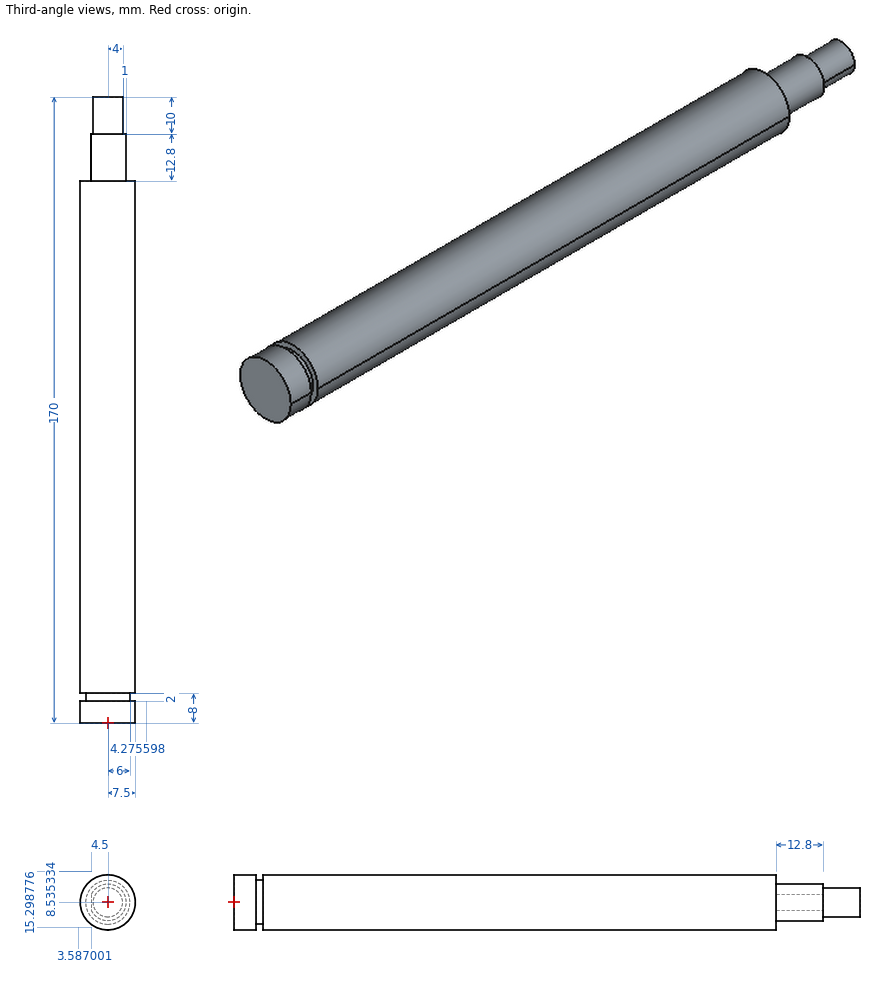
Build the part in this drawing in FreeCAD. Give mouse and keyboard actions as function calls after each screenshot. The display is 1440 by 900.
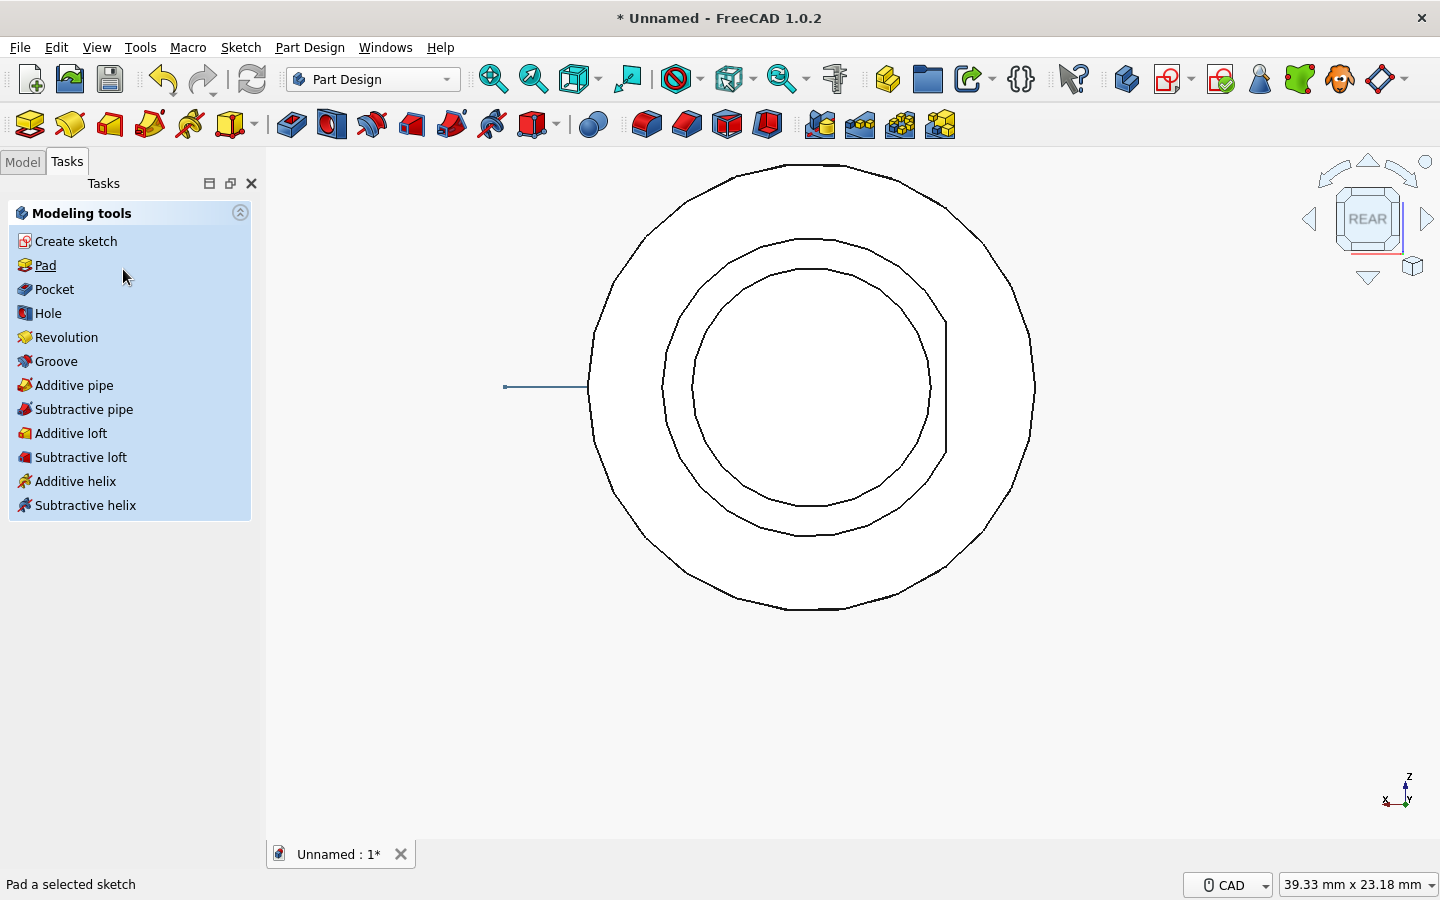
click(372, 124)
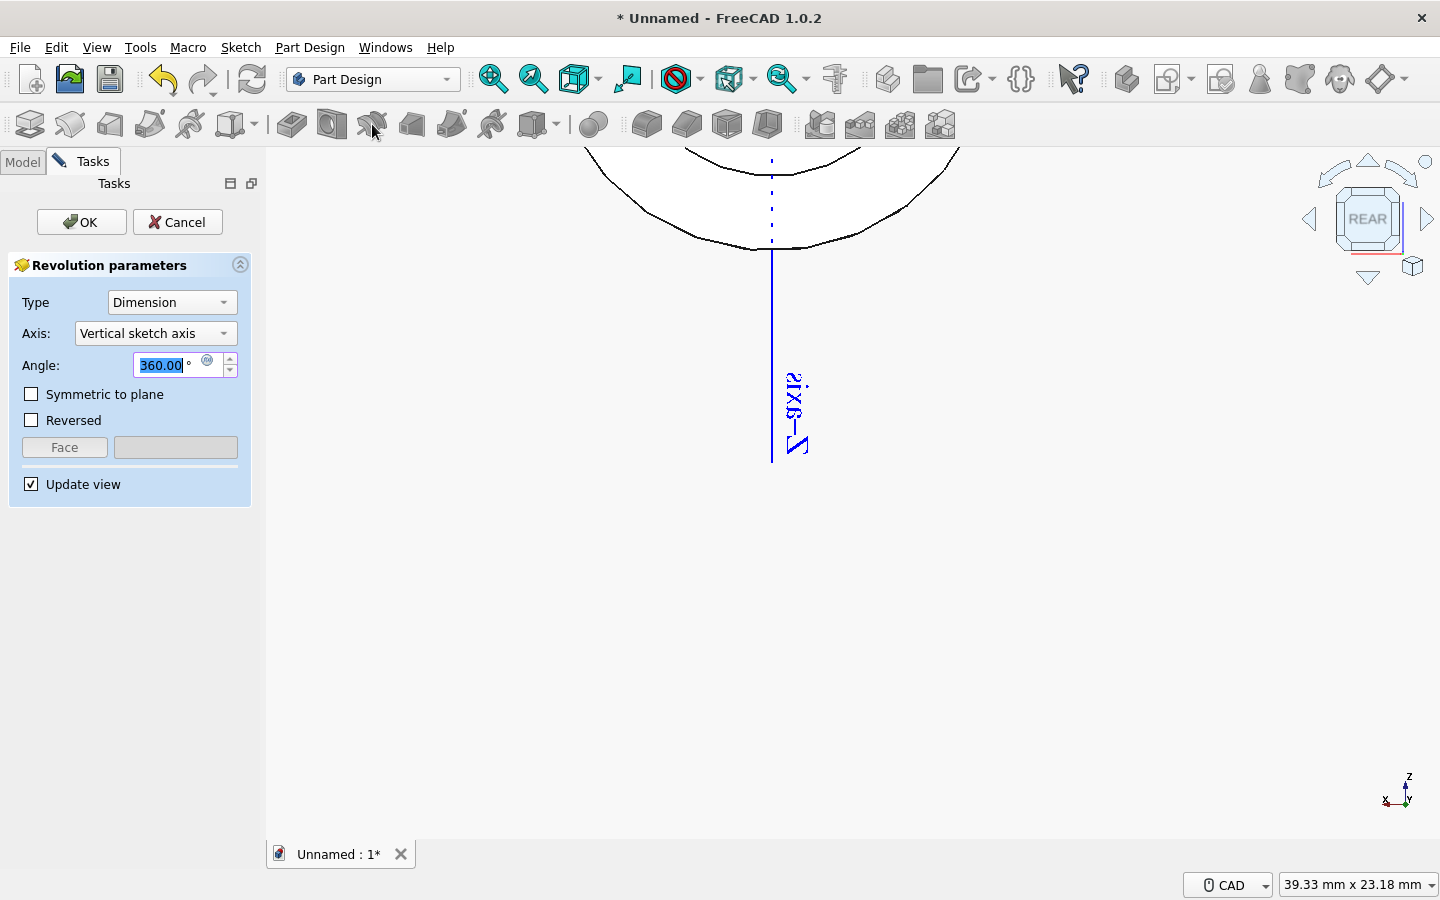
click(82, 222)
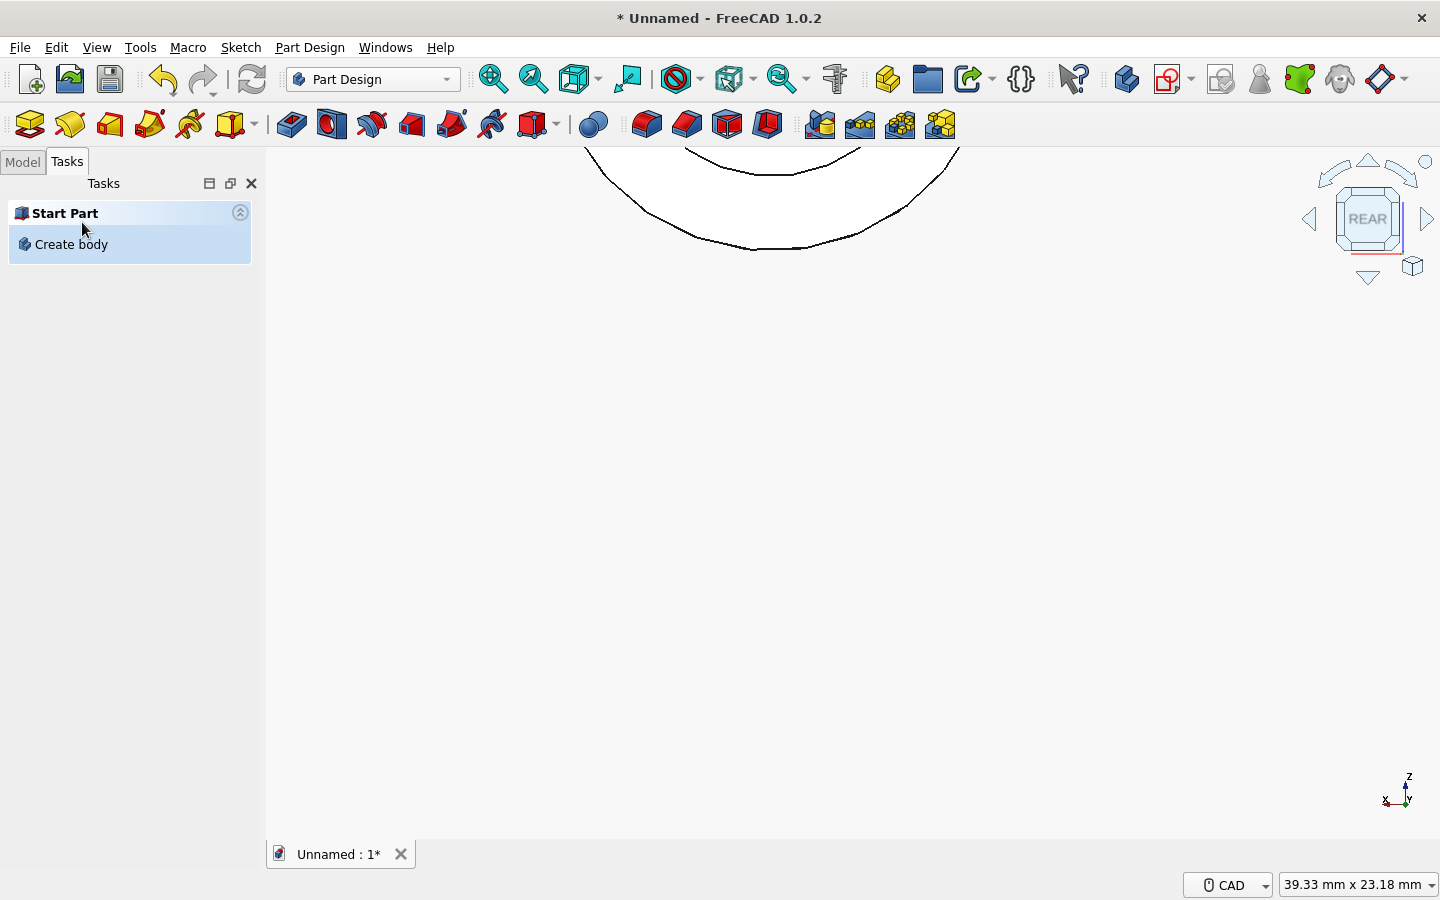
key(0)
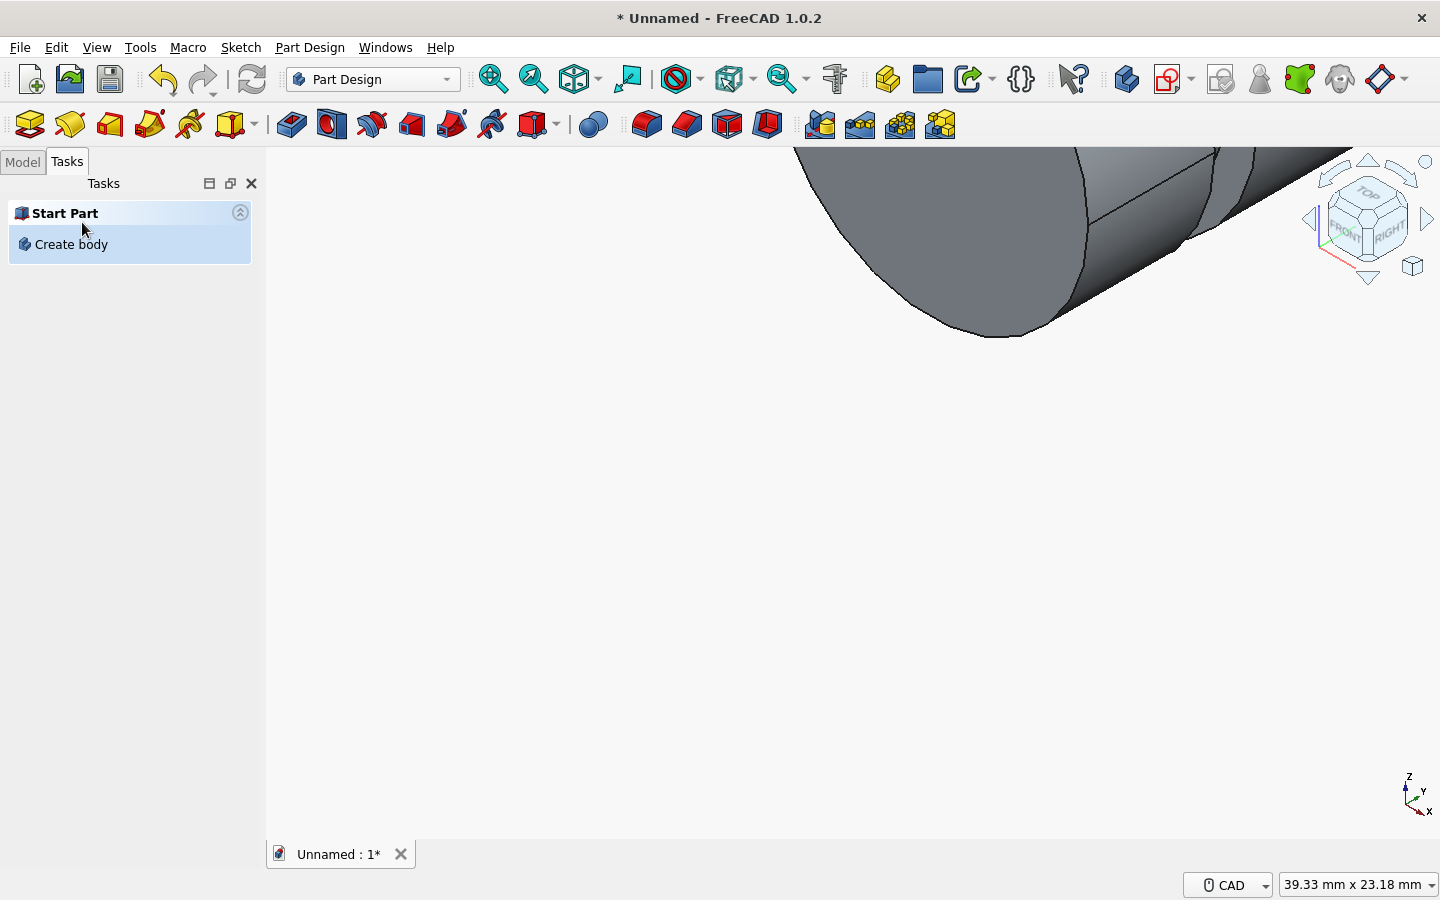
click(494, 80)